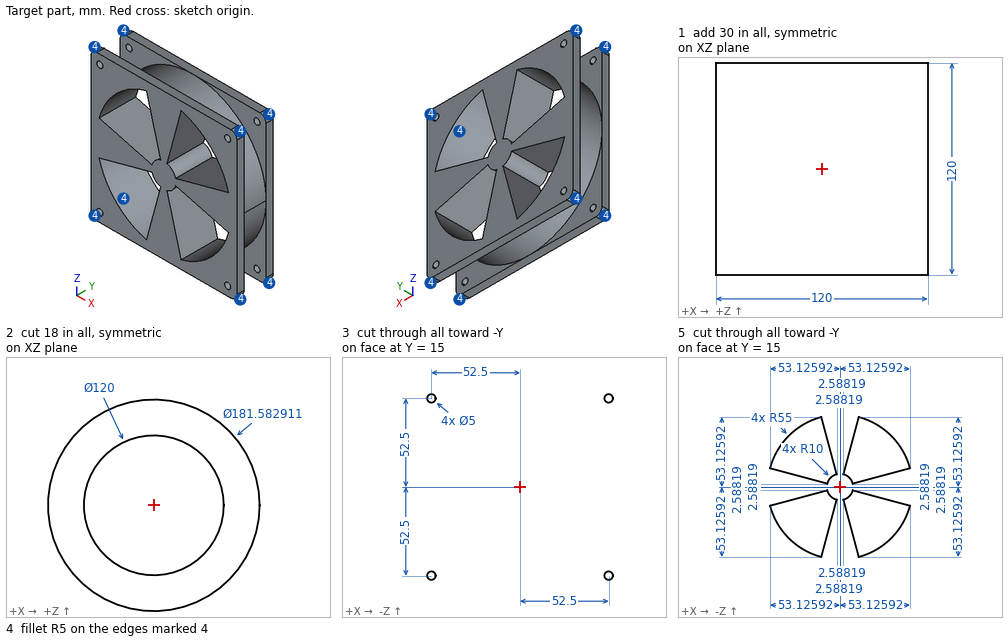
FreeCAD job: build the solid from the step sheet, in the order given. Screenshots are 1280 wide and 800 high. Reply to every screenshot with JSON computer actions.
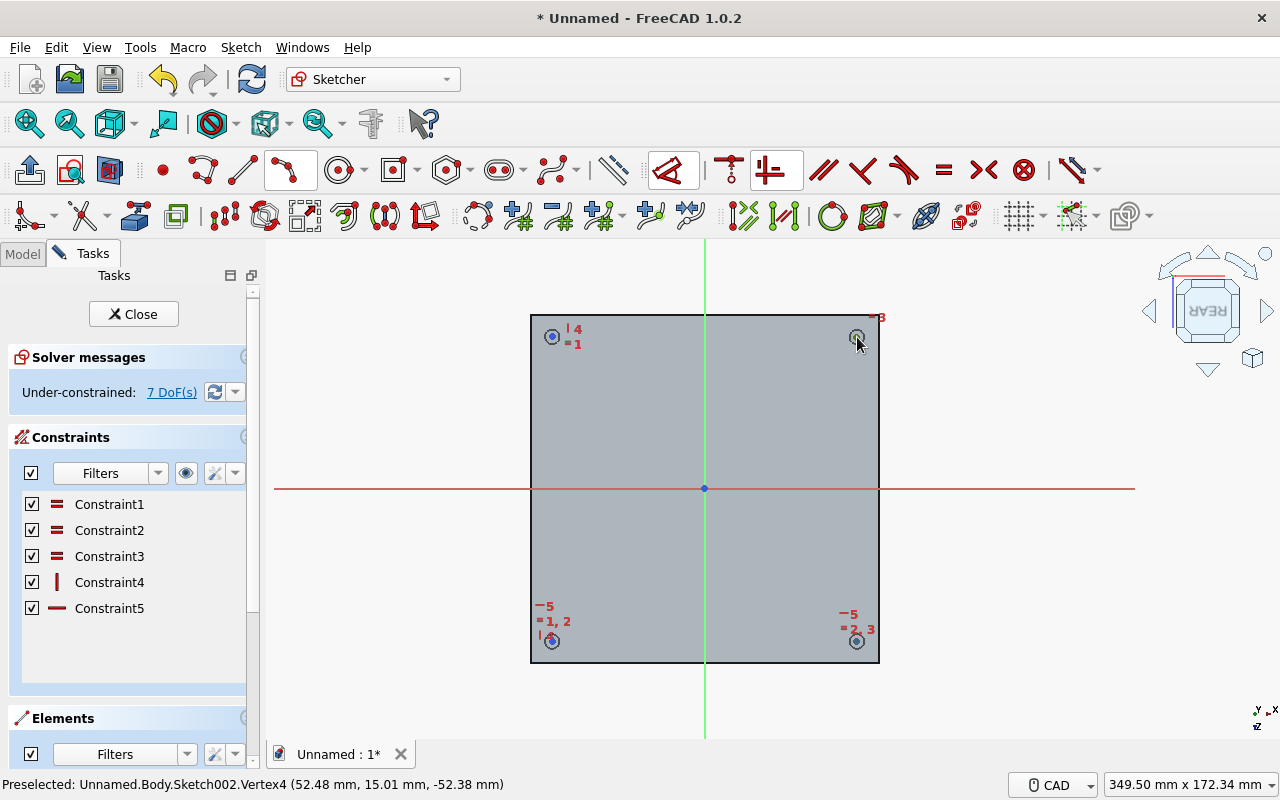
{"action": "left_click", "coordinate": [798, 170]}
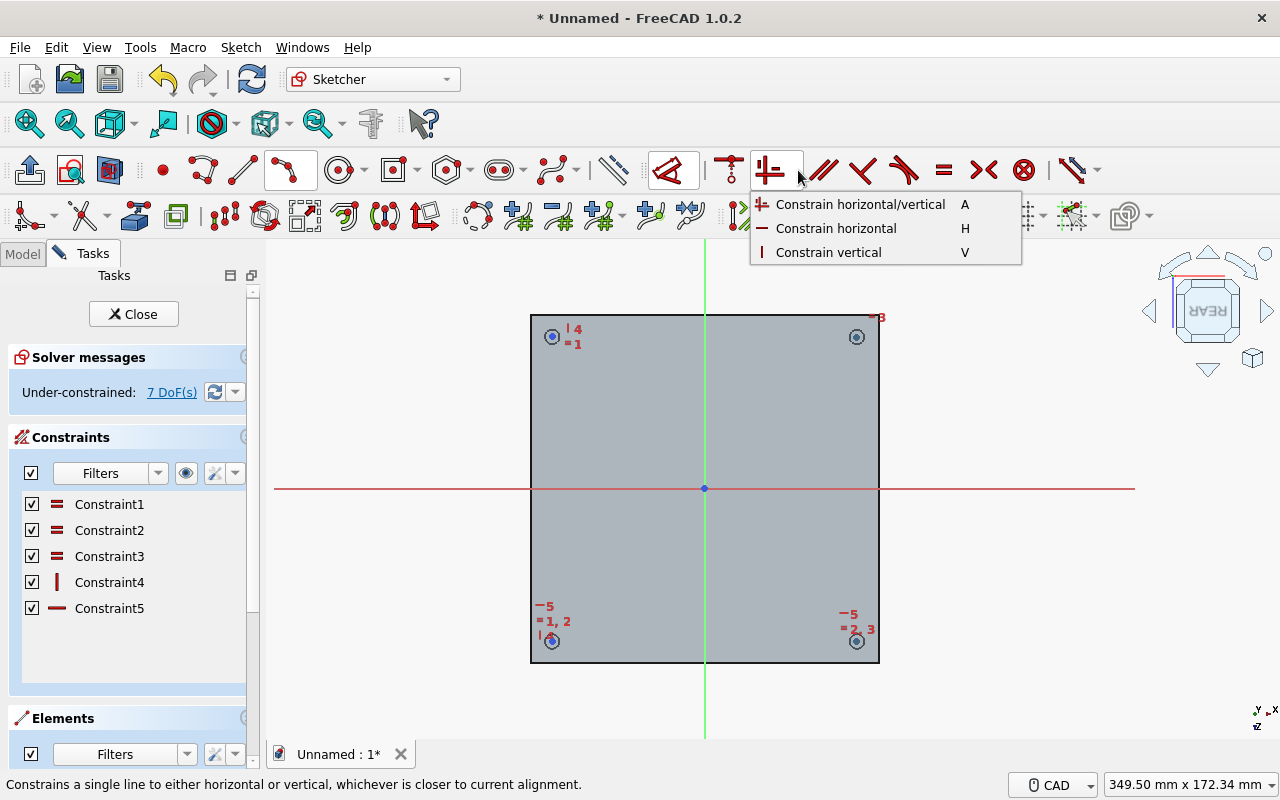
{"action": "left_click", "coordinate": [886, 252]}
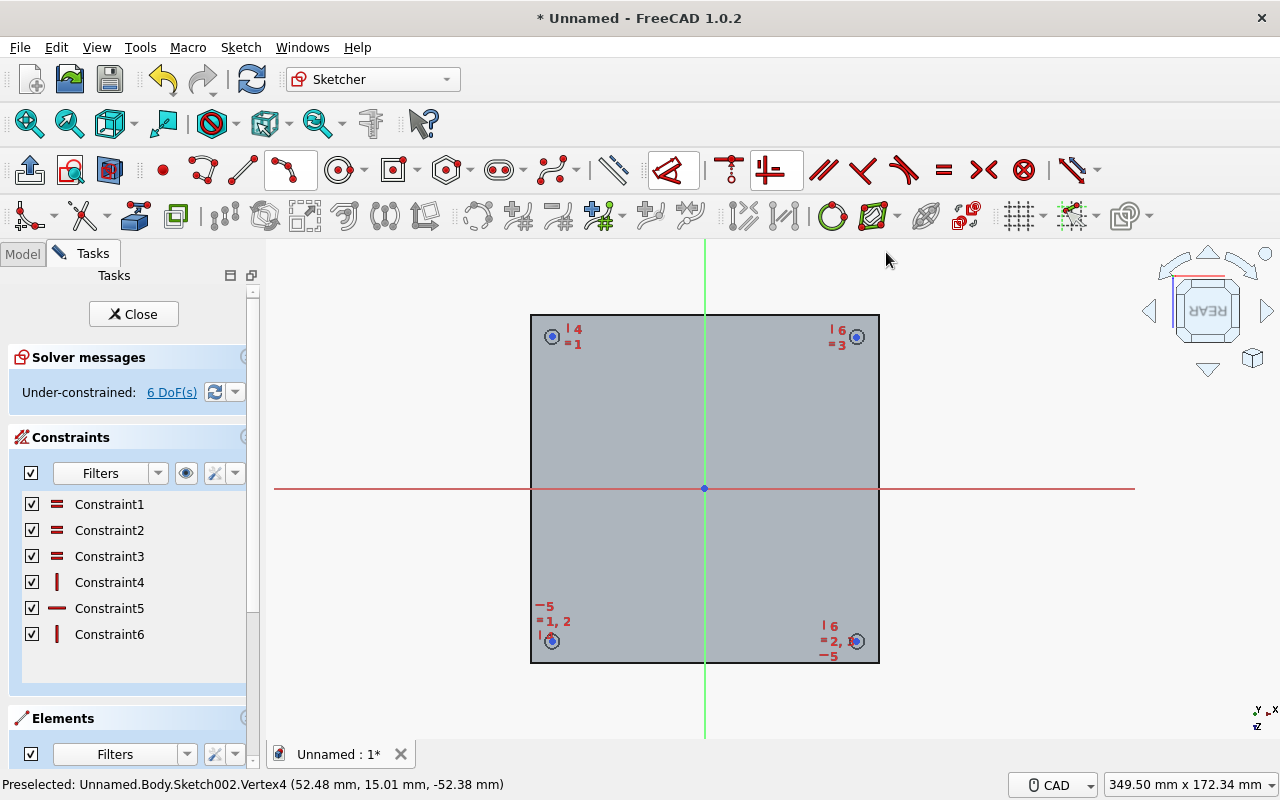
{"action": "left_click", "coordinate": [552, 337]}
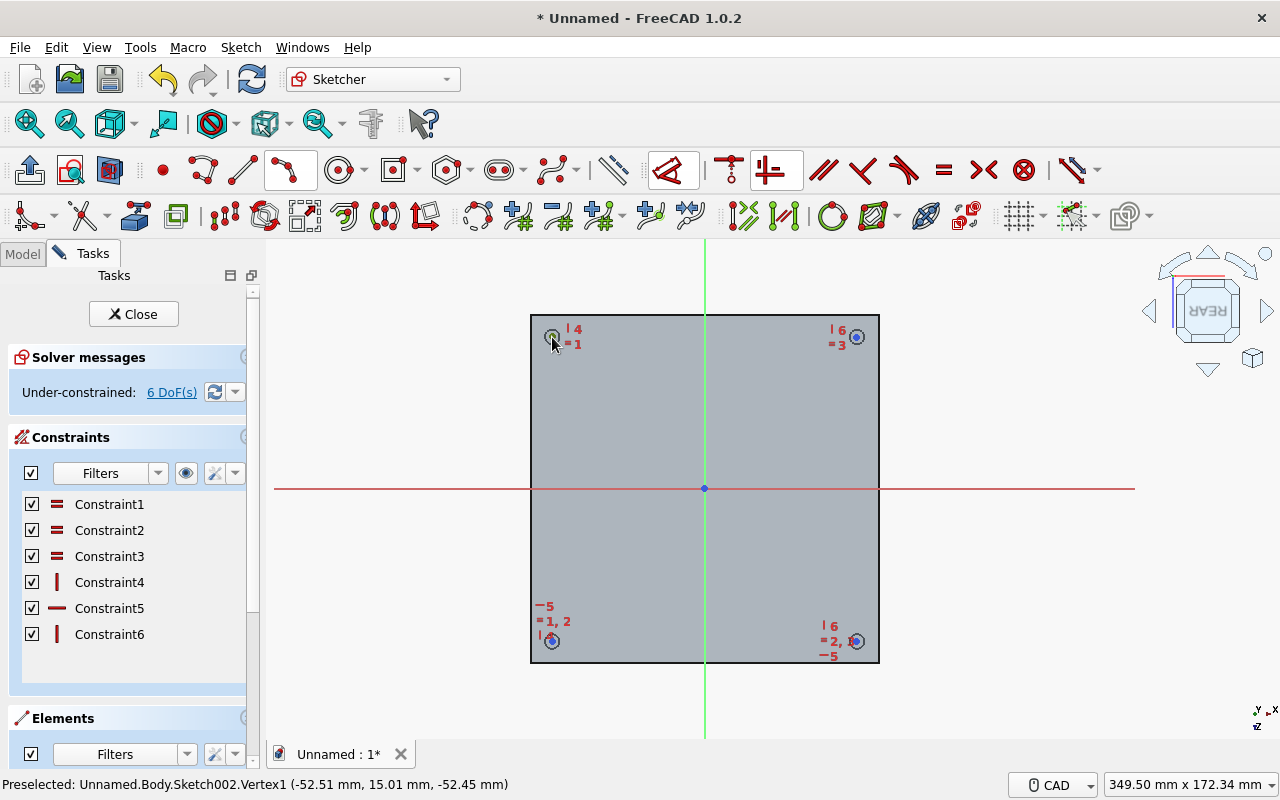
{"action": "left_click", "coordinate": [857, 337]}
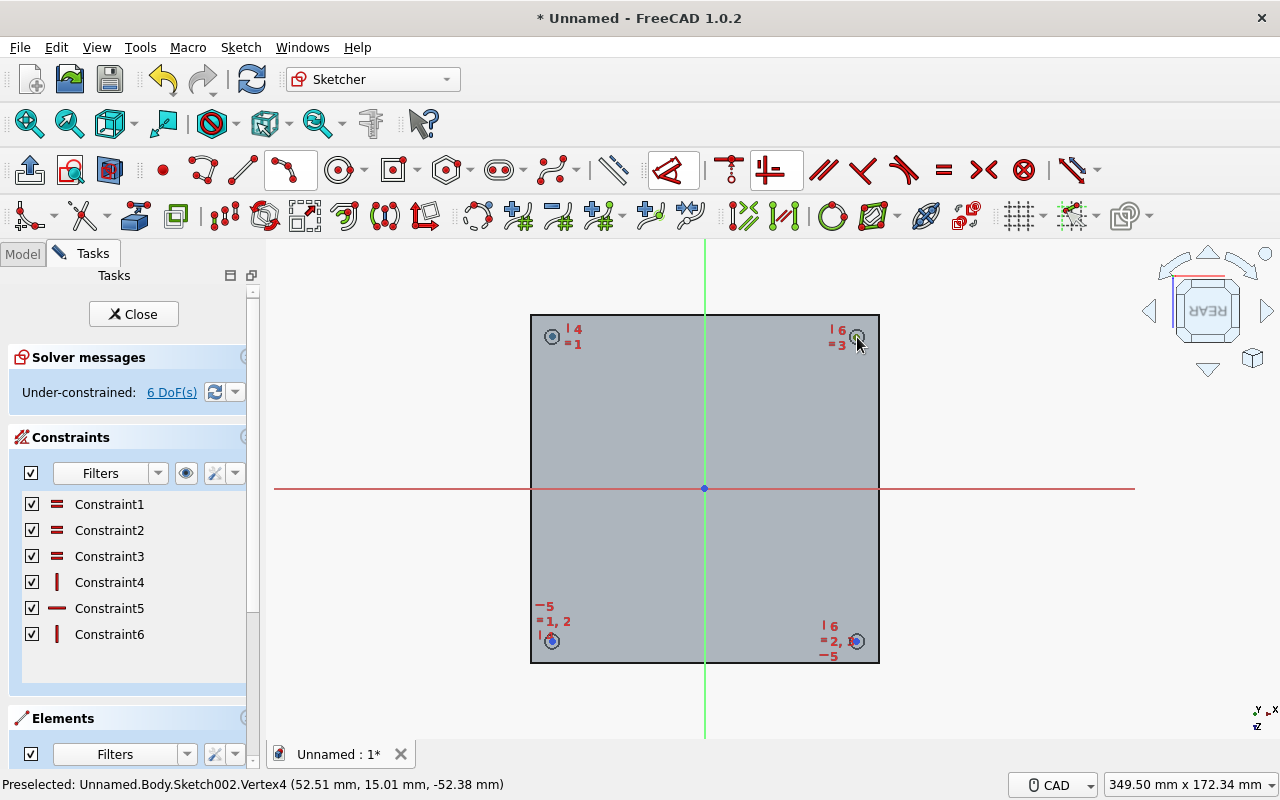
{"action": "left_click", "coordinate": [798, 170]}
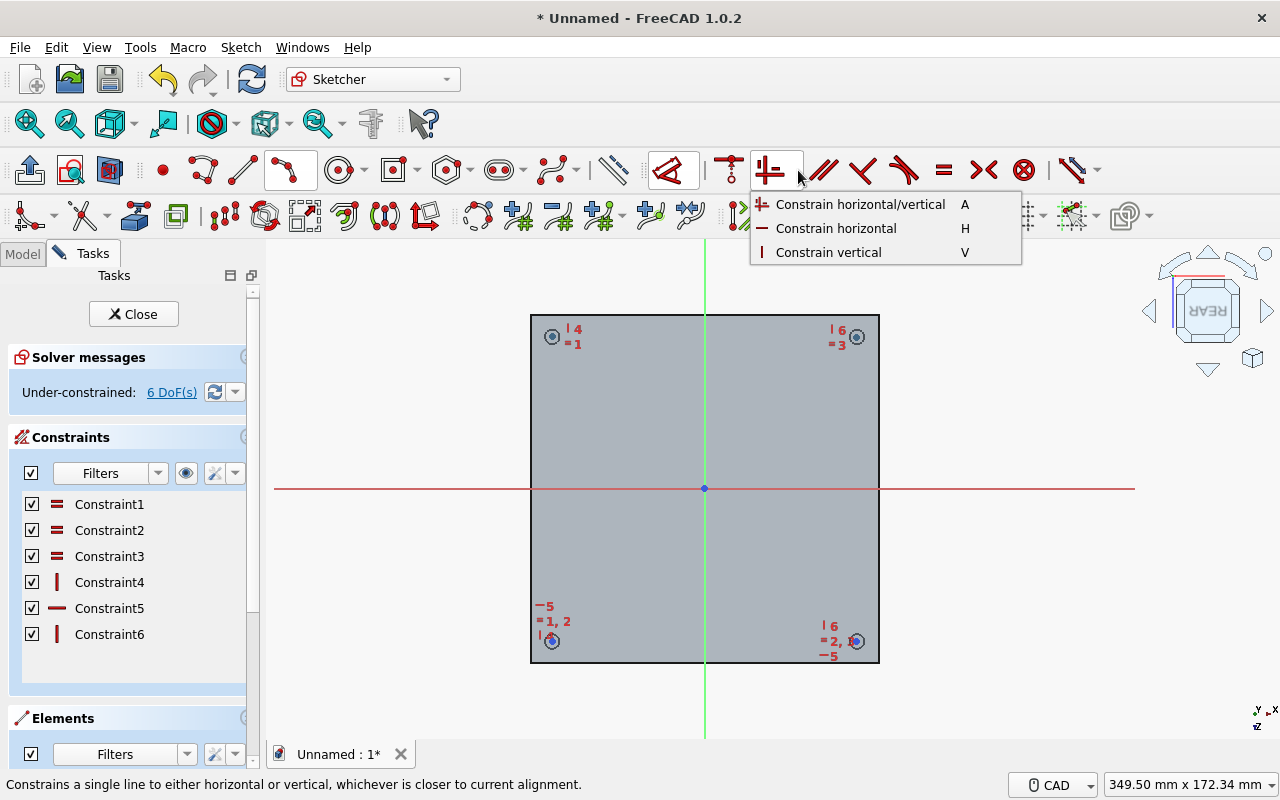
{"action": "left_click", "coordinate": [886, 228]}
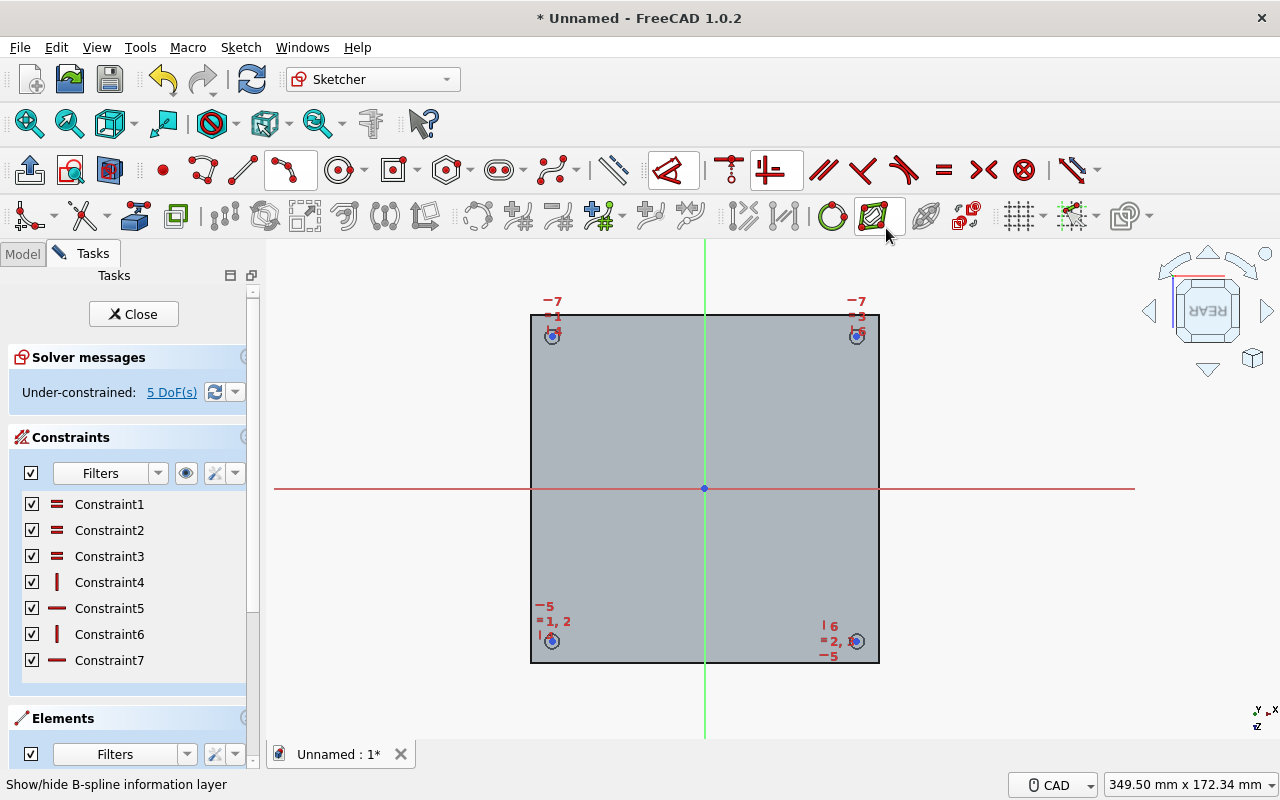
{"action": "scroll", "coordinate": [552, 330], "scroll_direction": "up", "scroll_amount": 6}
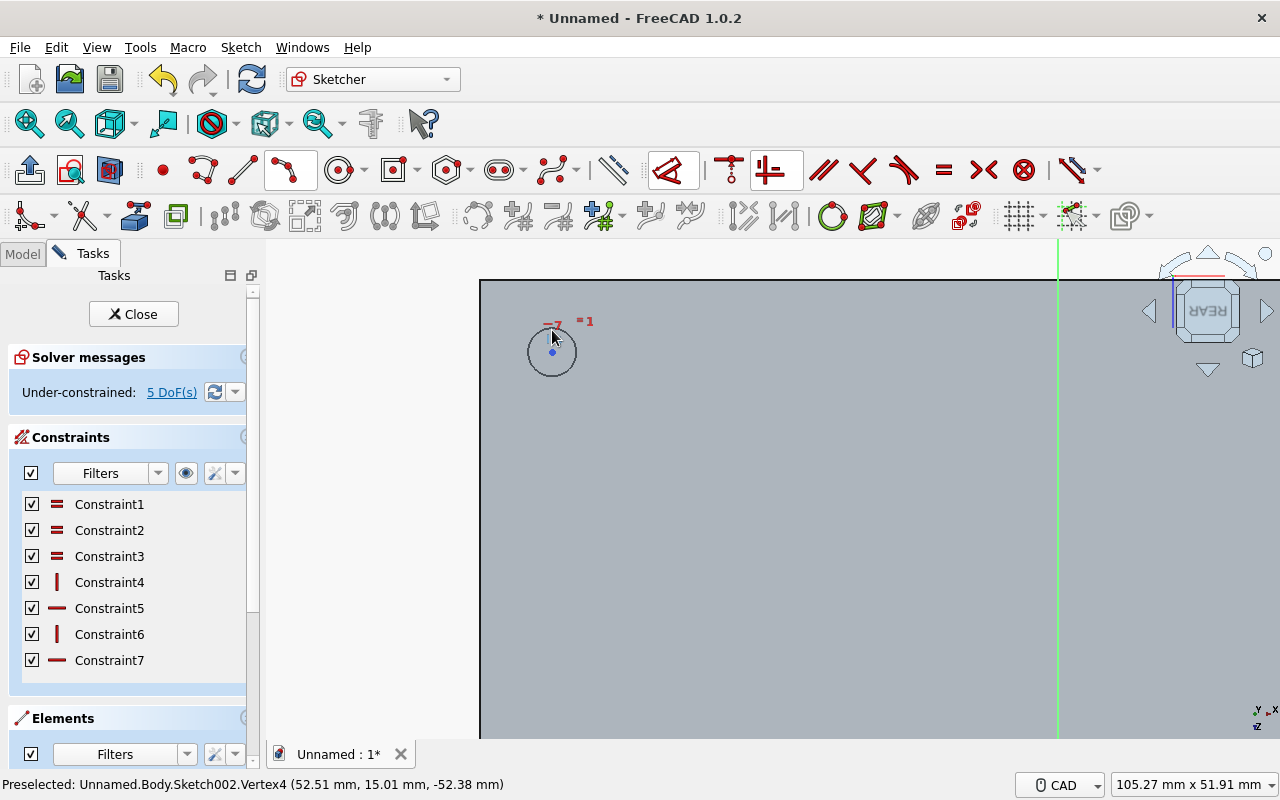
{"action": "left_click", "coordinate": [528, 352]}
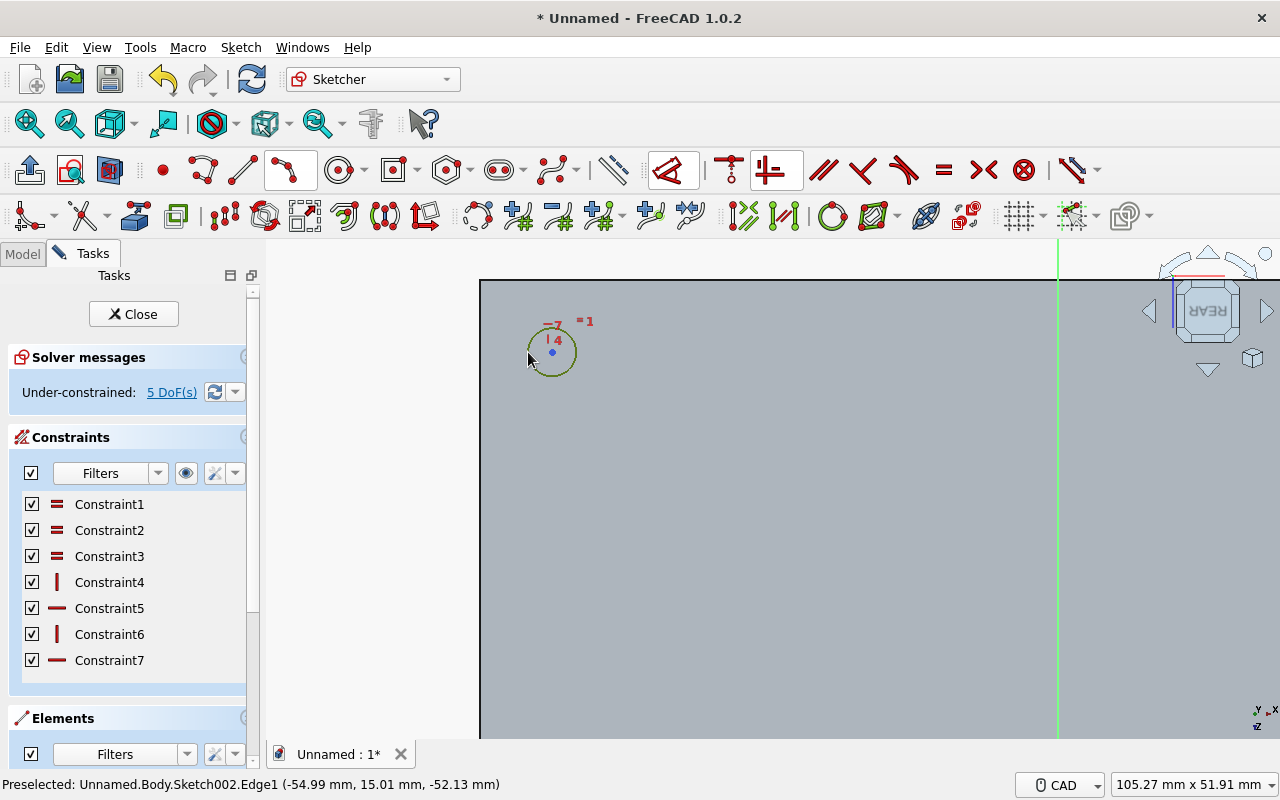
{"action": "key", "text": "k o"}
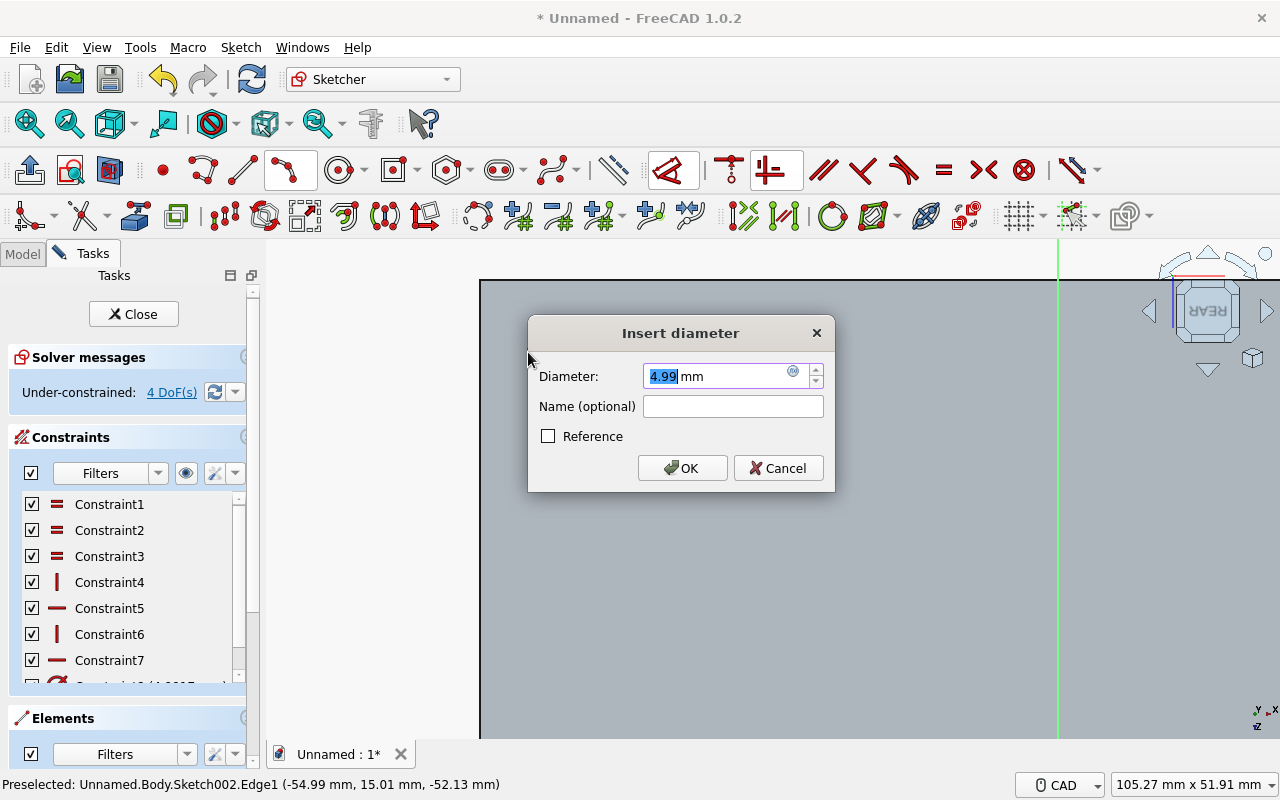
{"action": "type", "text": "5"}
{"action": "key", "text": "Return"}